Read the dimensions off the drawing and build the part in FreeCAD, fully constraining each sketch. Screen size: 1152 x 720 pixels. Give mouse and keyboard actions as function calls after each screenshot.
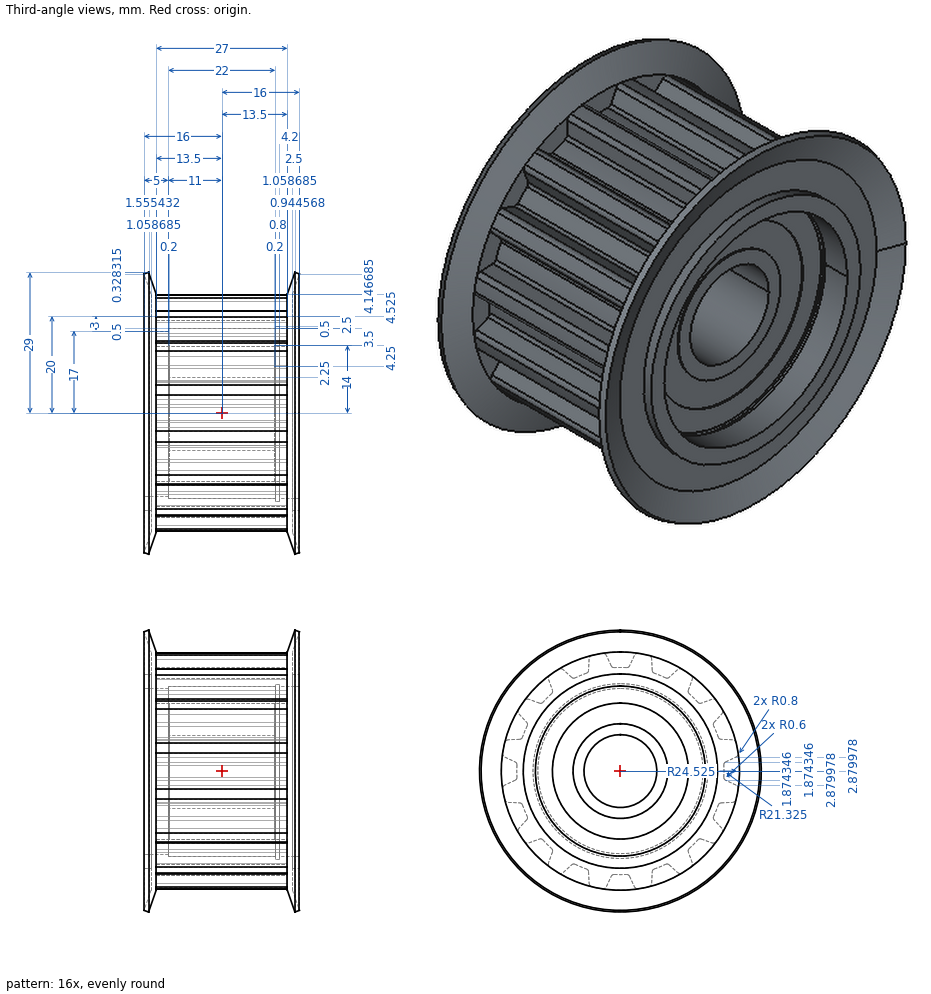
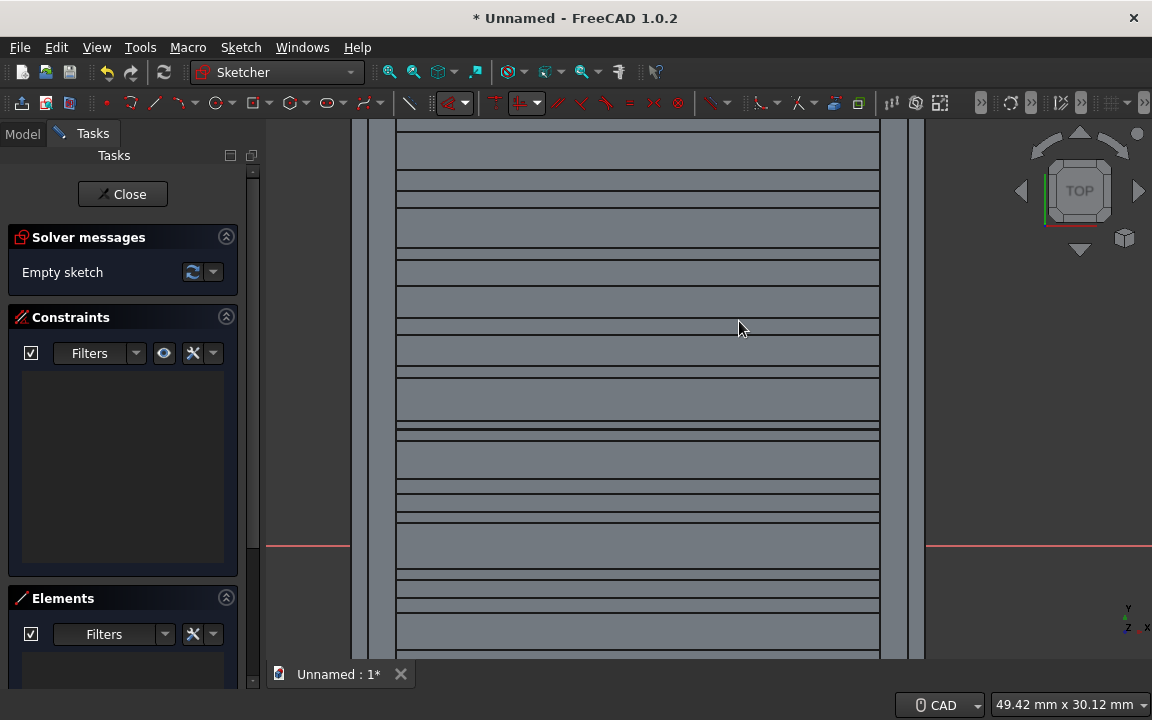
click(132, 104)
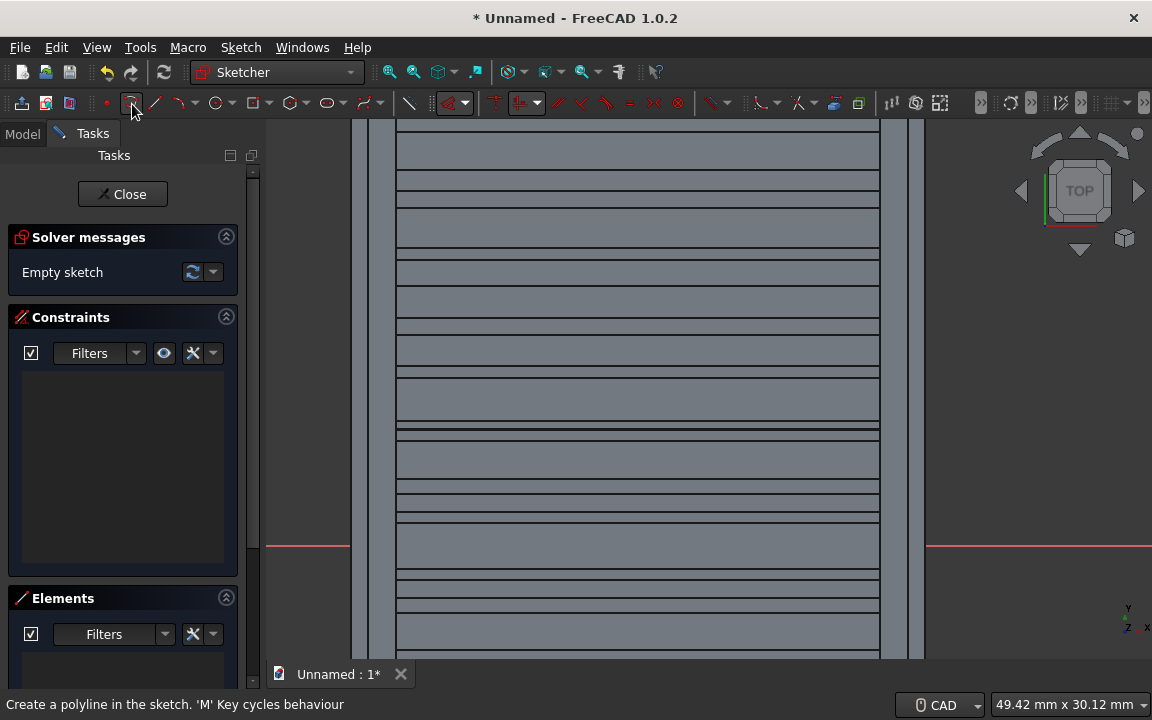
click(441, 411)
click(835, 411)
click(835, 371)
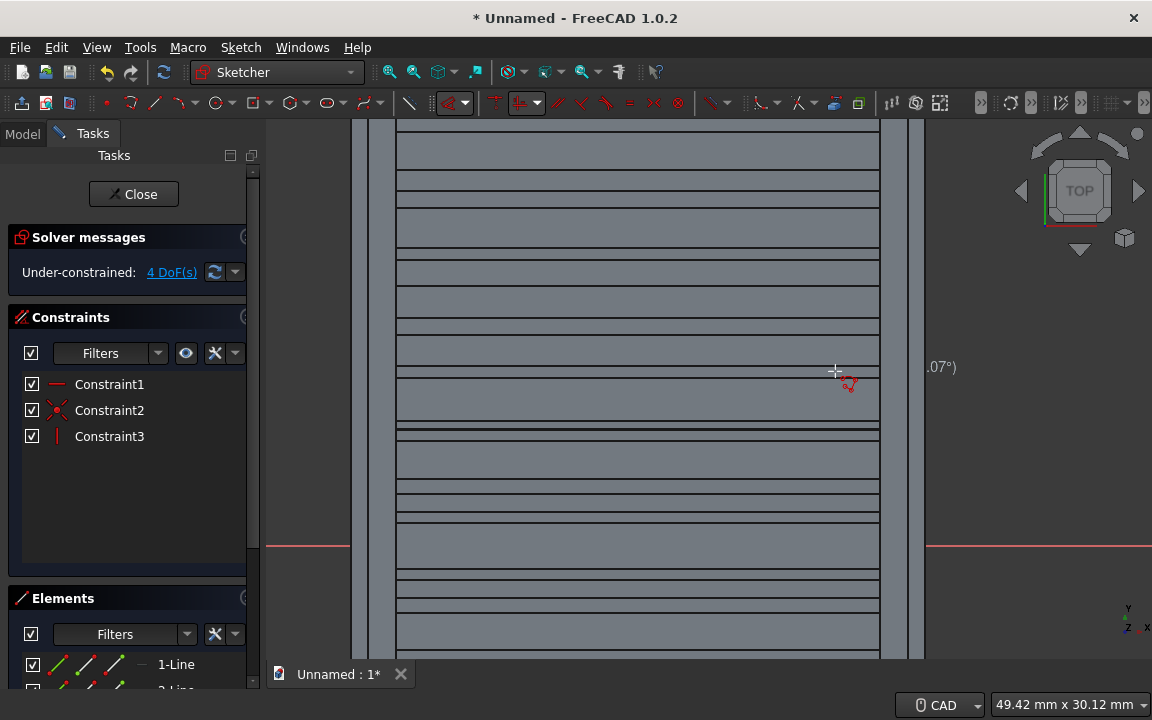
scroll(832, 371, up, 8)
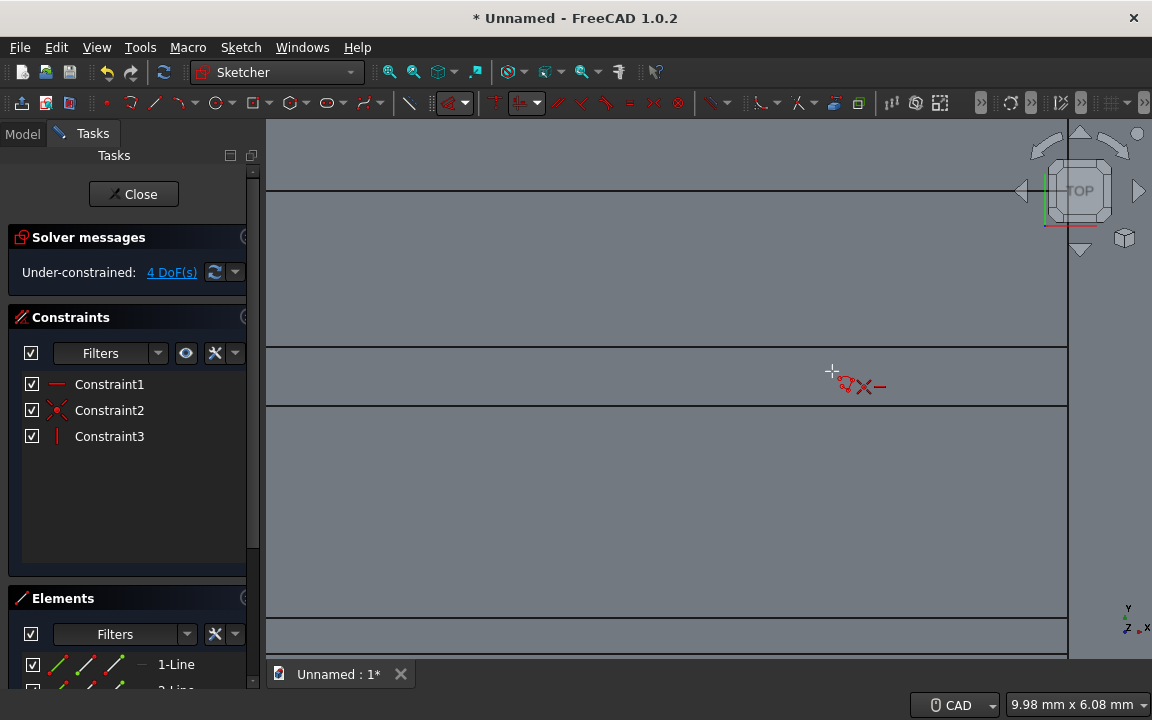
click(828, 369)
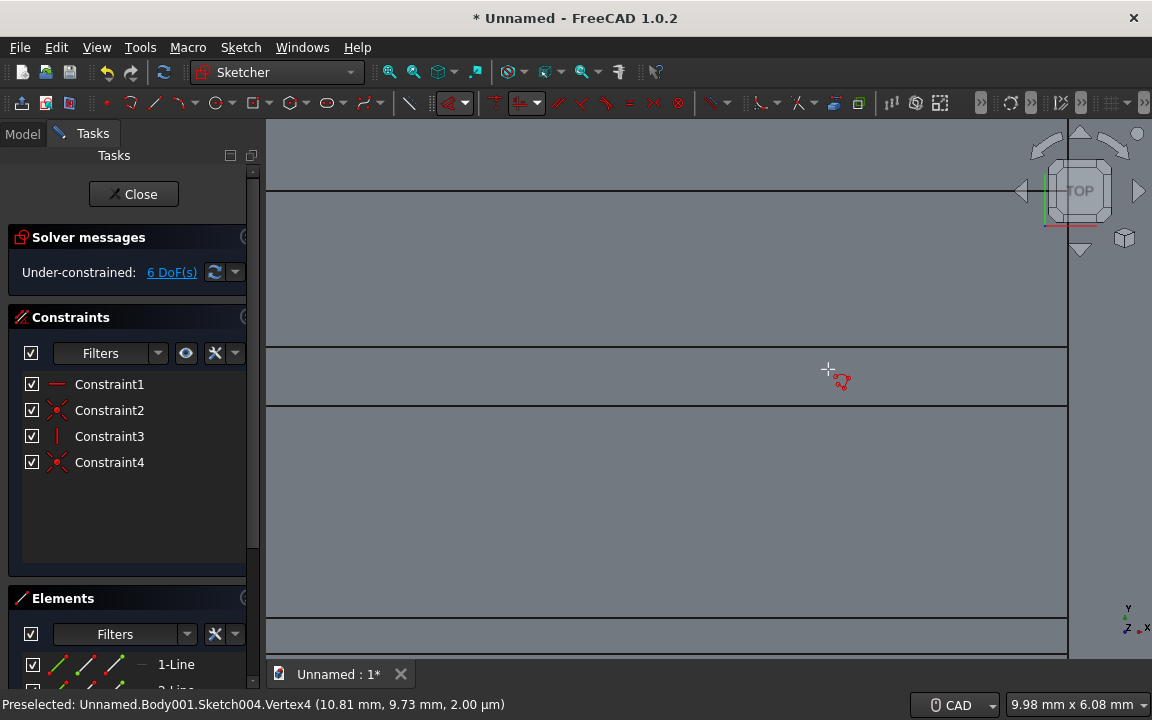
scroll(836, 371, down, 8)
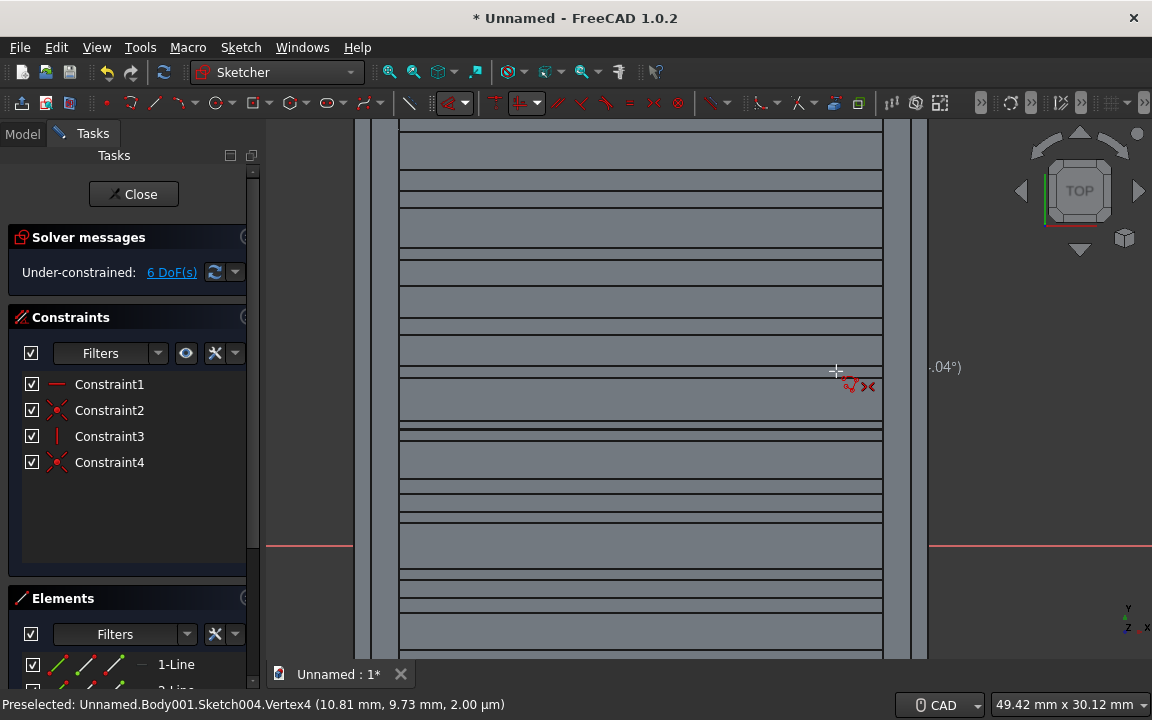
click(835, 295)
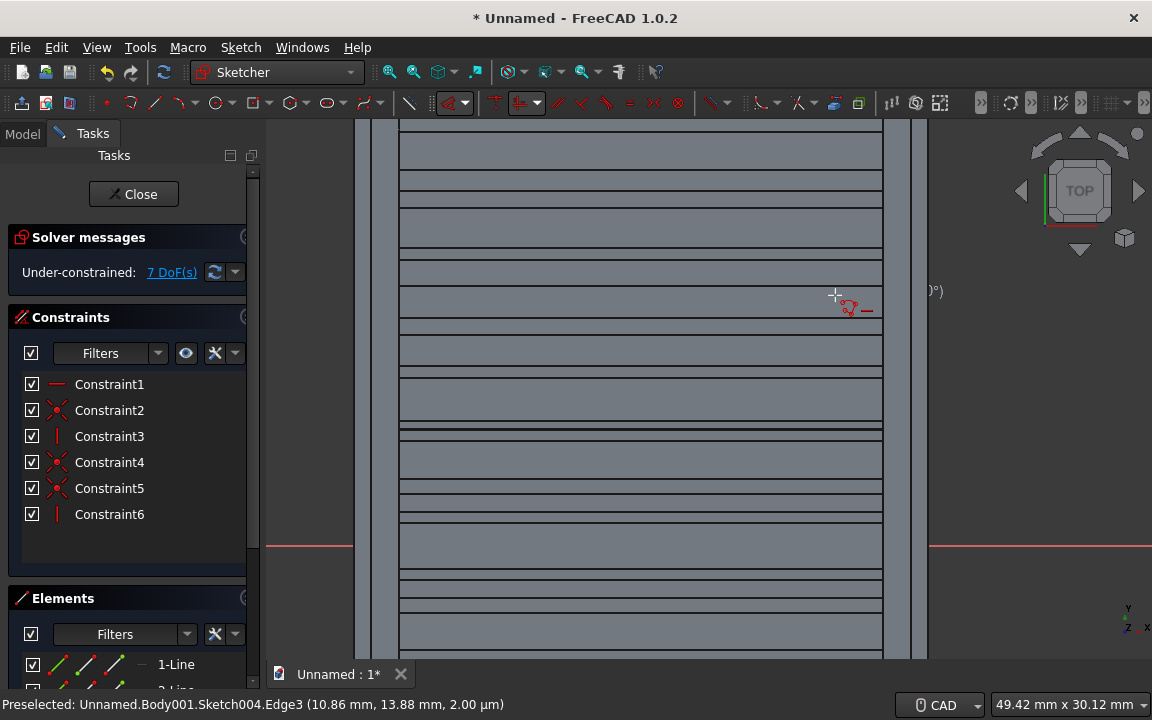
scroll(839, 295, up, 8)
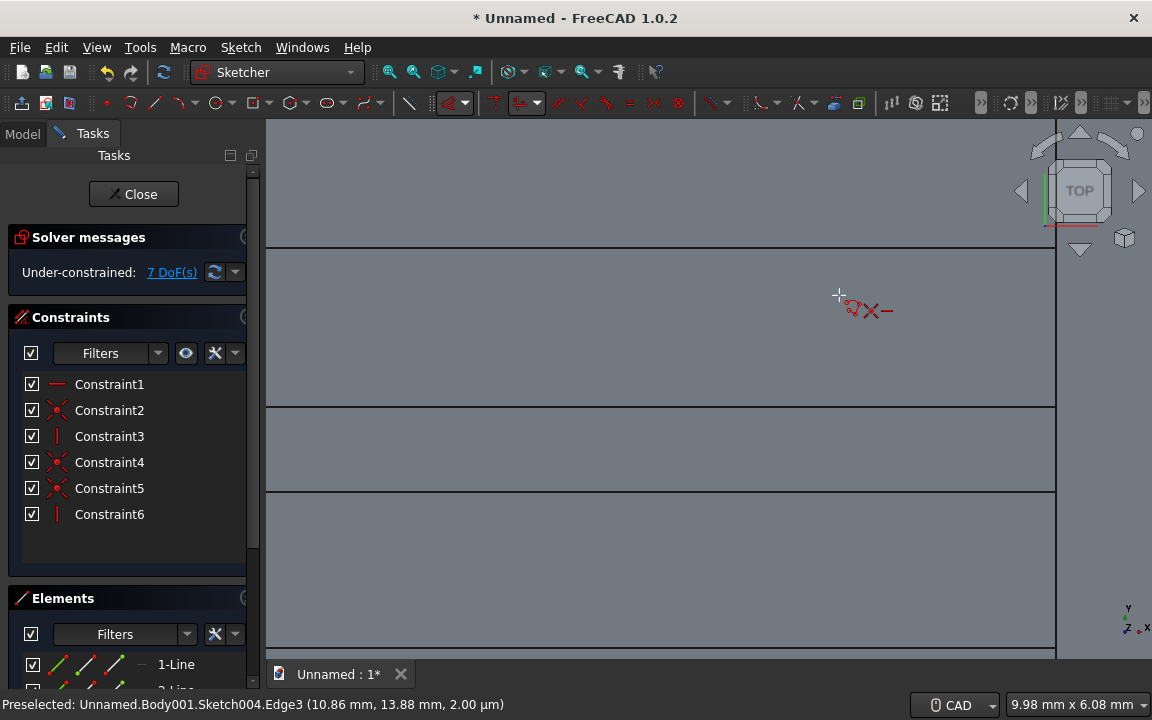
click(834, 294)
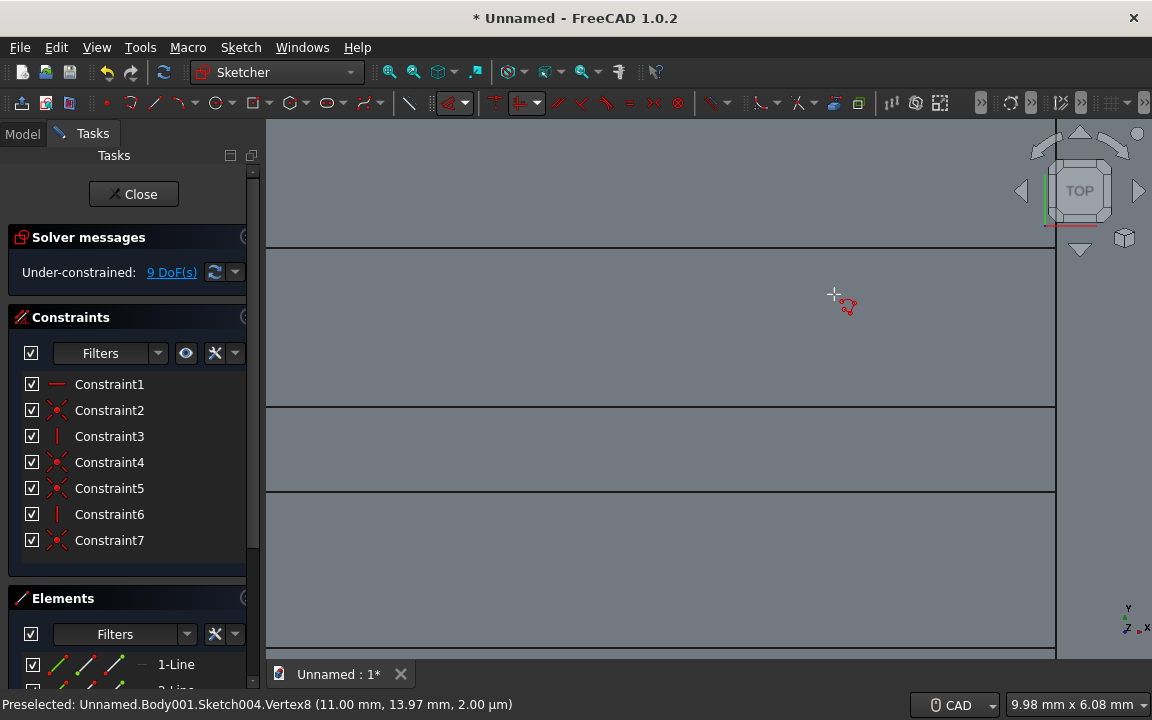
scroll(839, 295, down, 8)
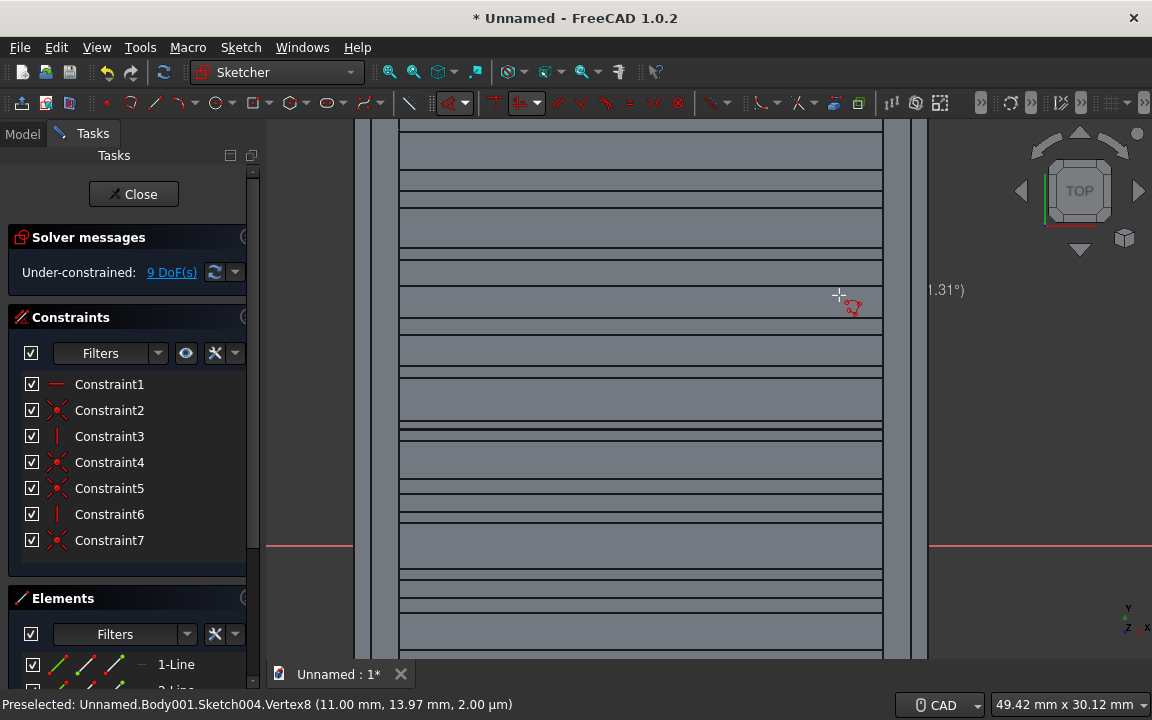
click(839, 232)
click(444, 232)
click(444, 295)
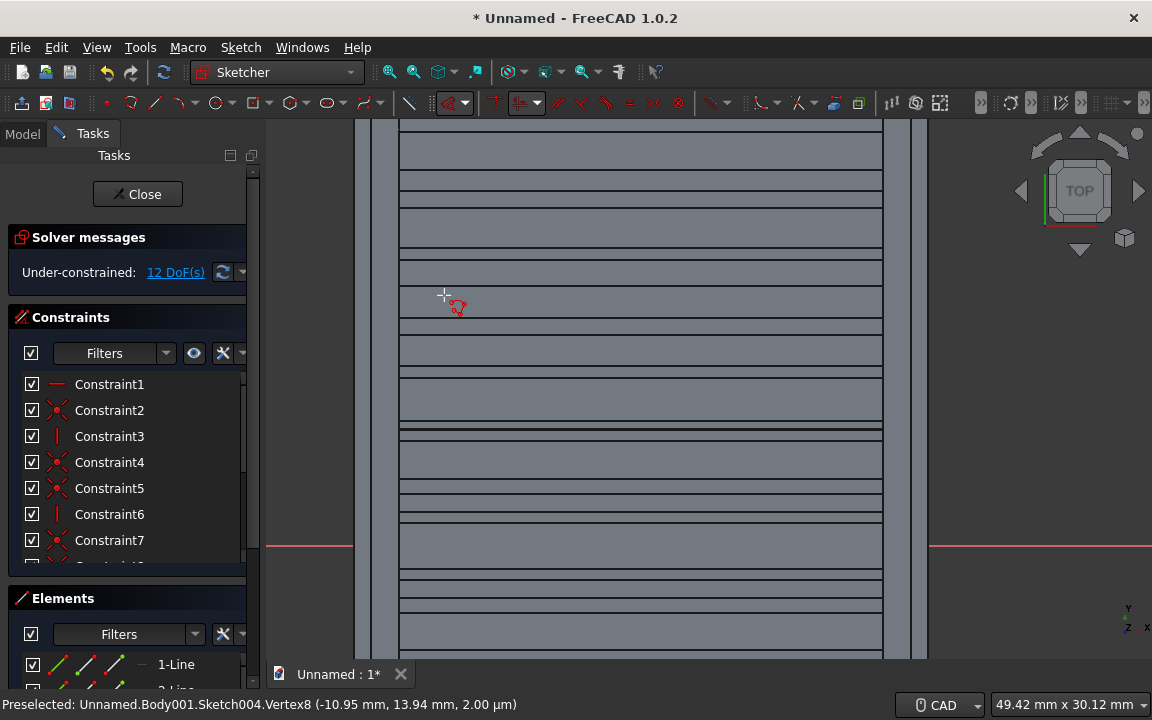
scroll(448, 295, up, 8)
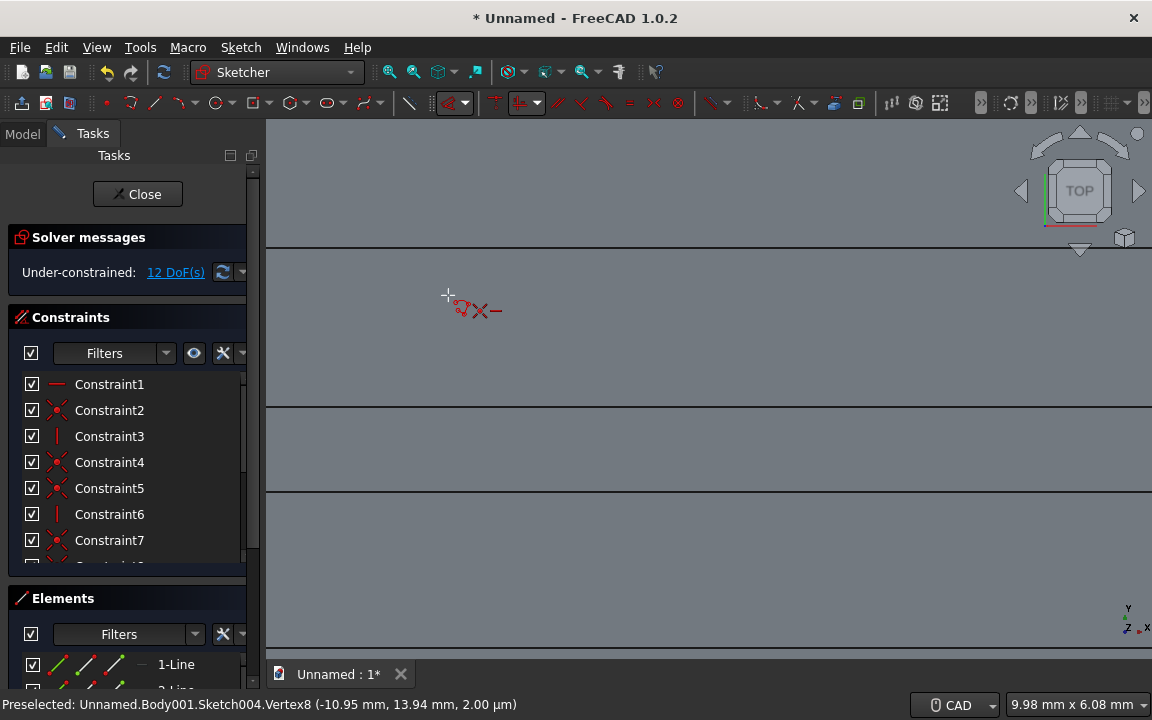
click(446, 294)